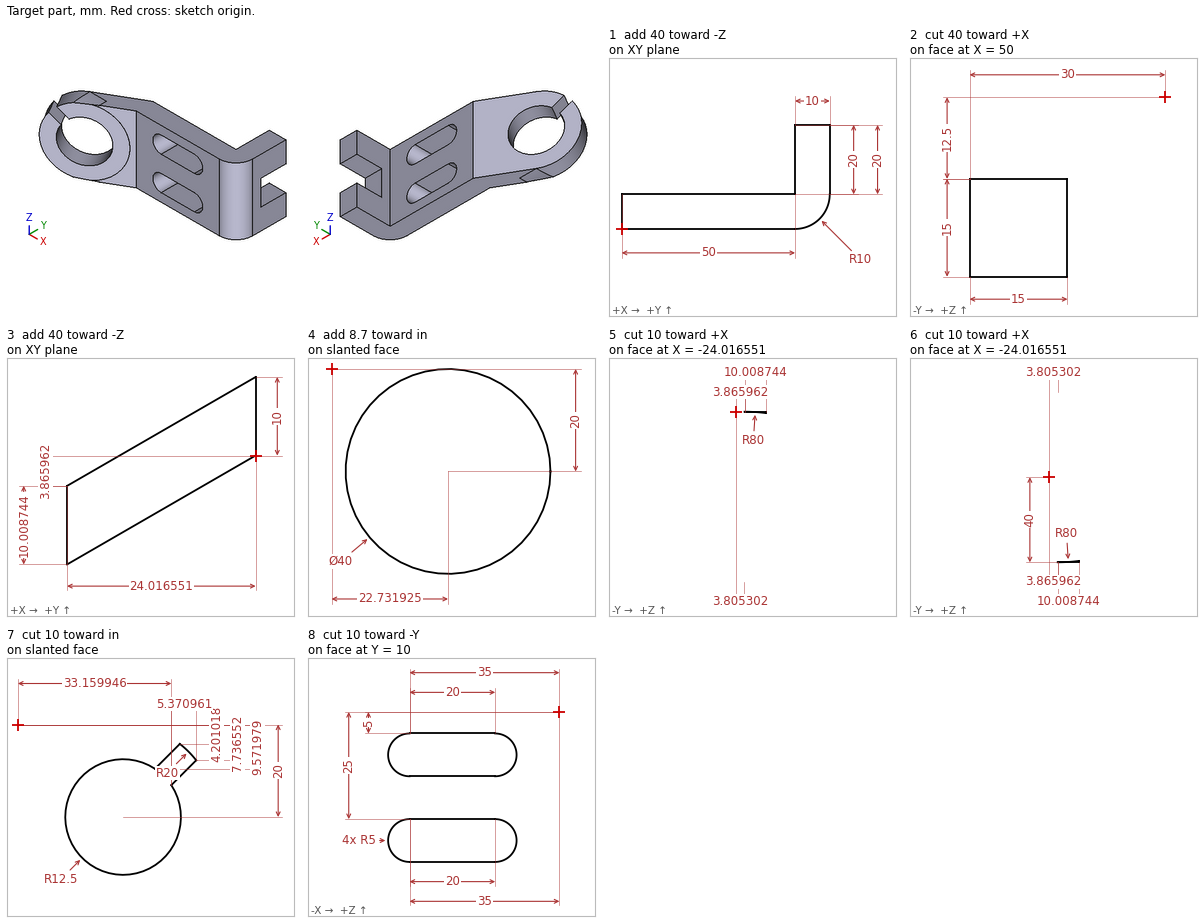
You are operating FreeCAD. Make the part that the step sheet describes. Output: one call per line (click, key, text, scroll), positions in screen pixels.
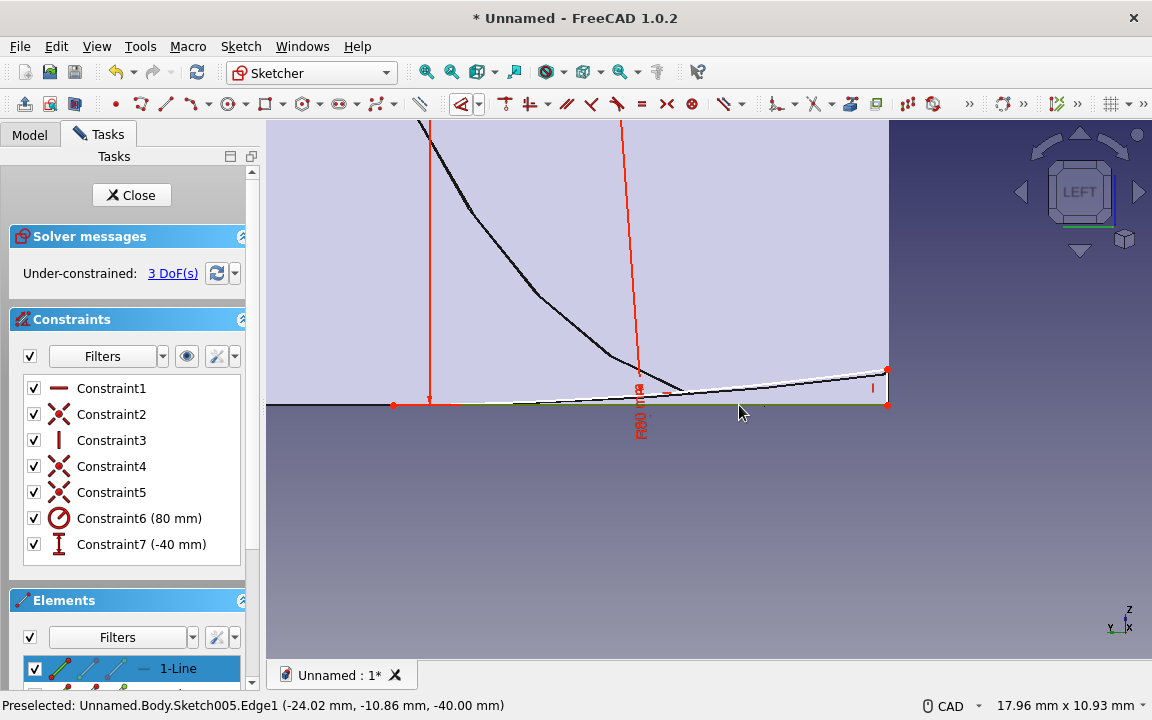
key(l)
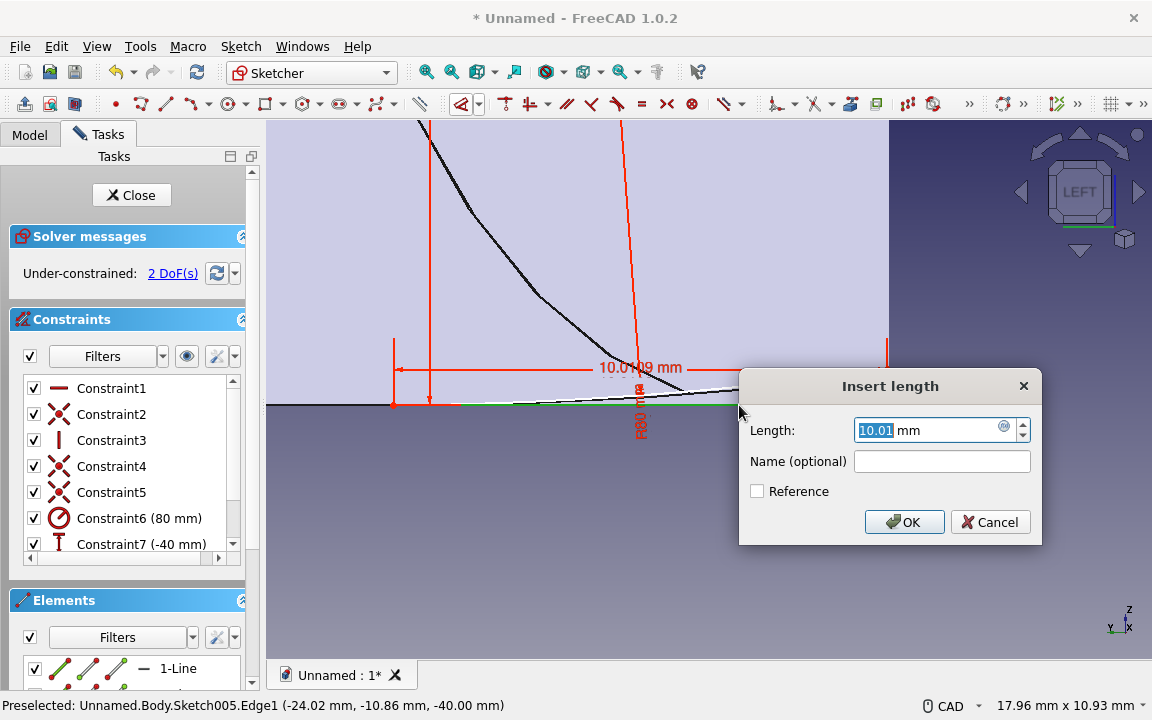
text(10.008744)
key(Return)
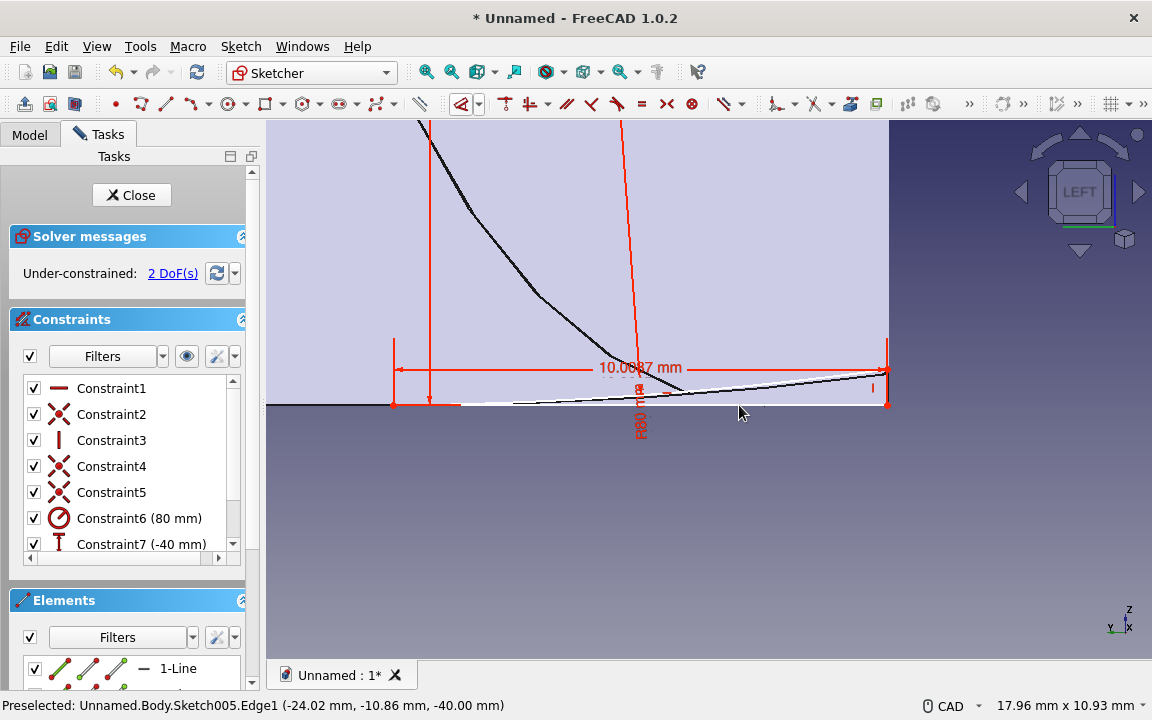
click(394, 405)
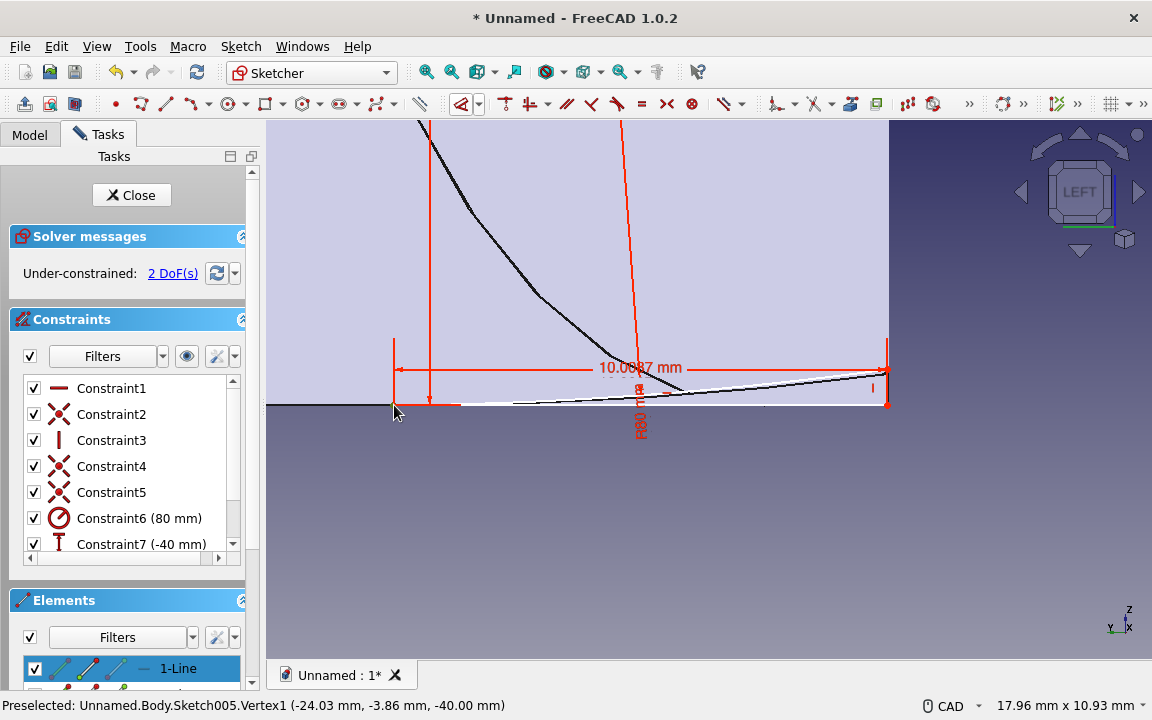
click(478, 104)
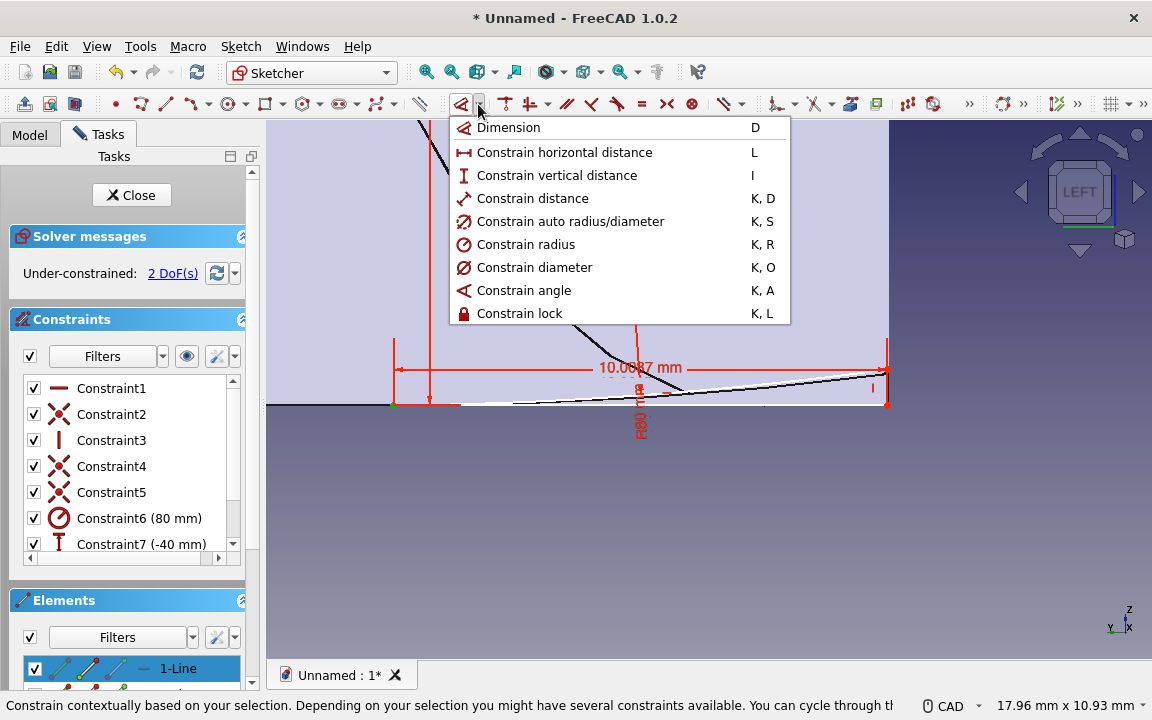
click(620, 152)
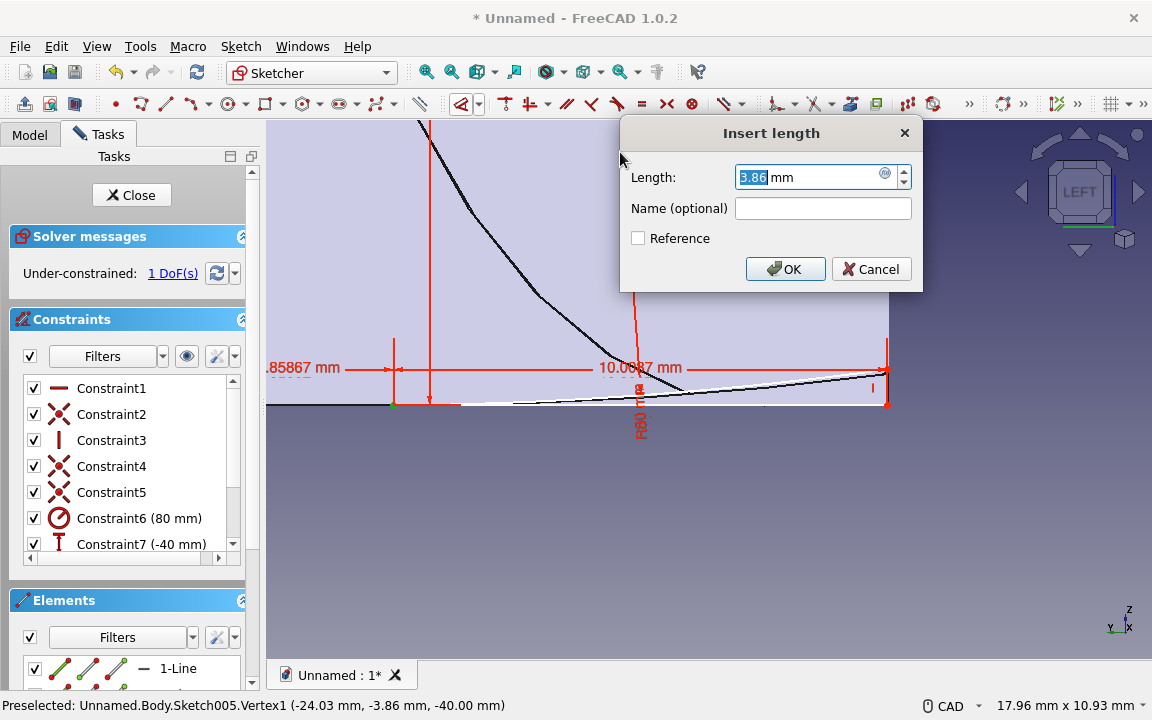
text(3.865962)
key(Return)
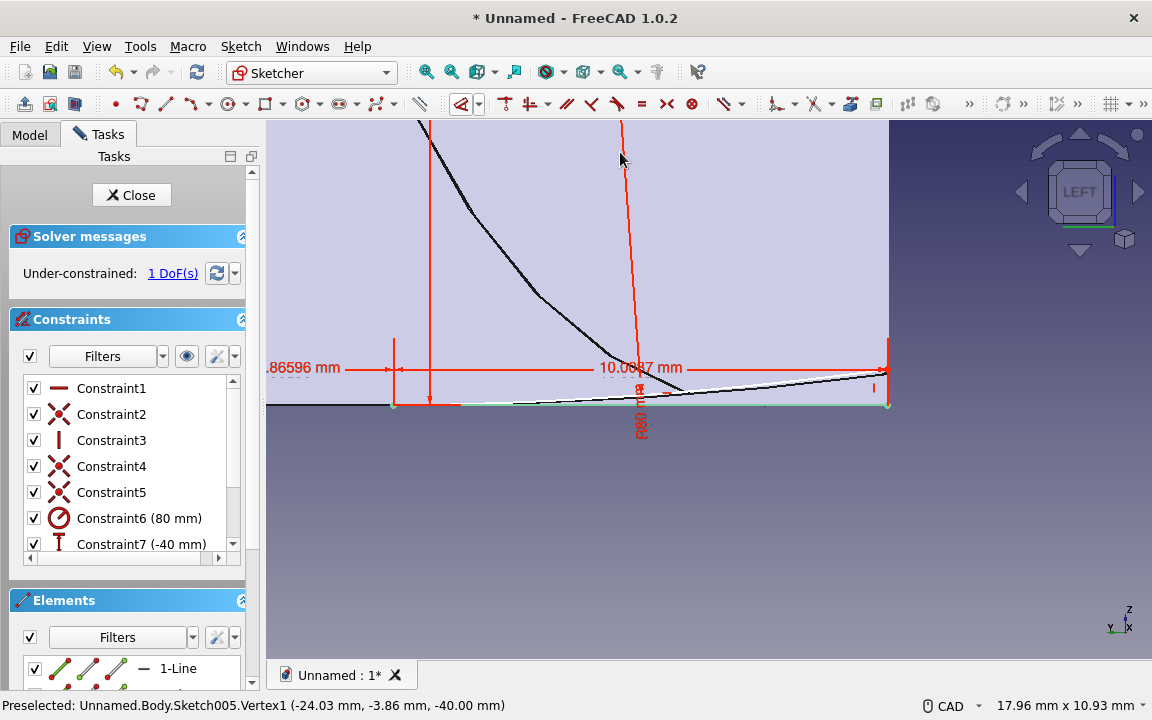
scroll(642, 585, down, 12)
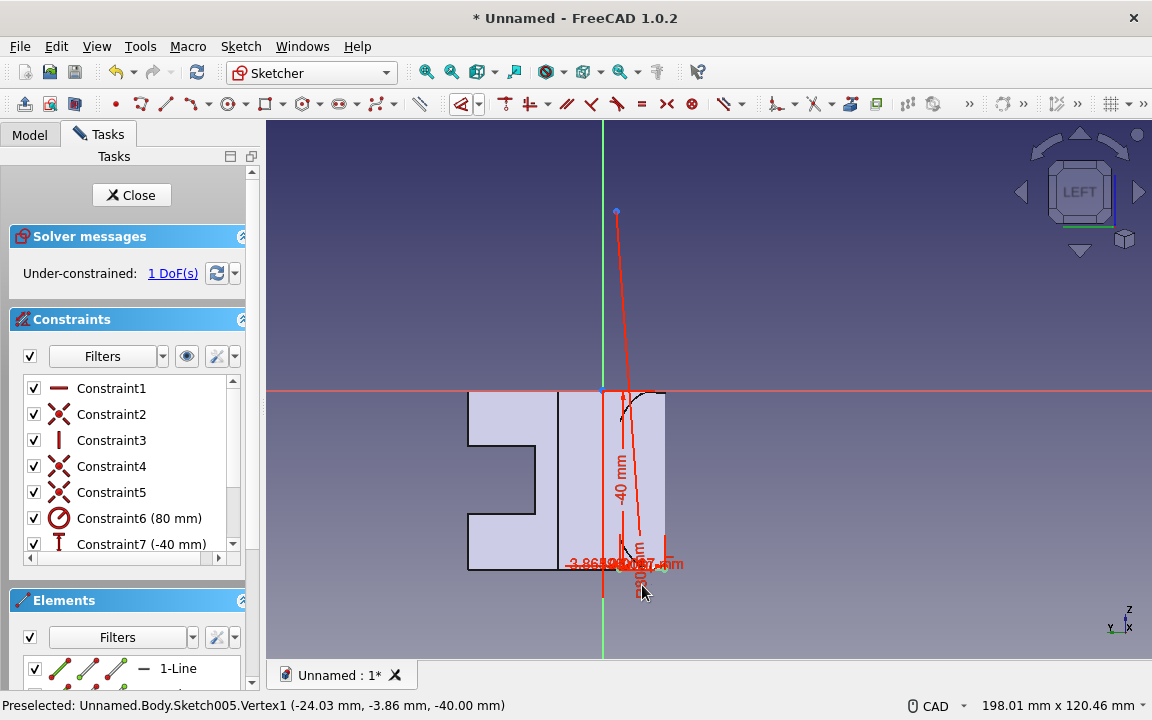
scroll(616, 212, up, 5)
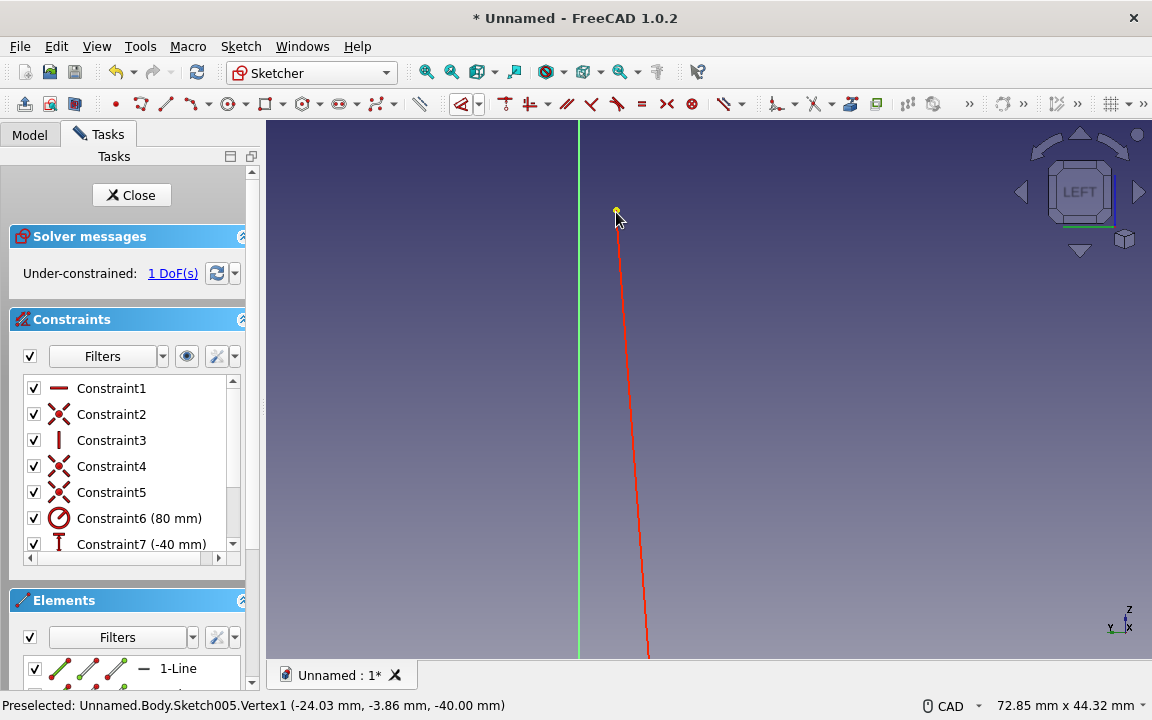
click(616, 211)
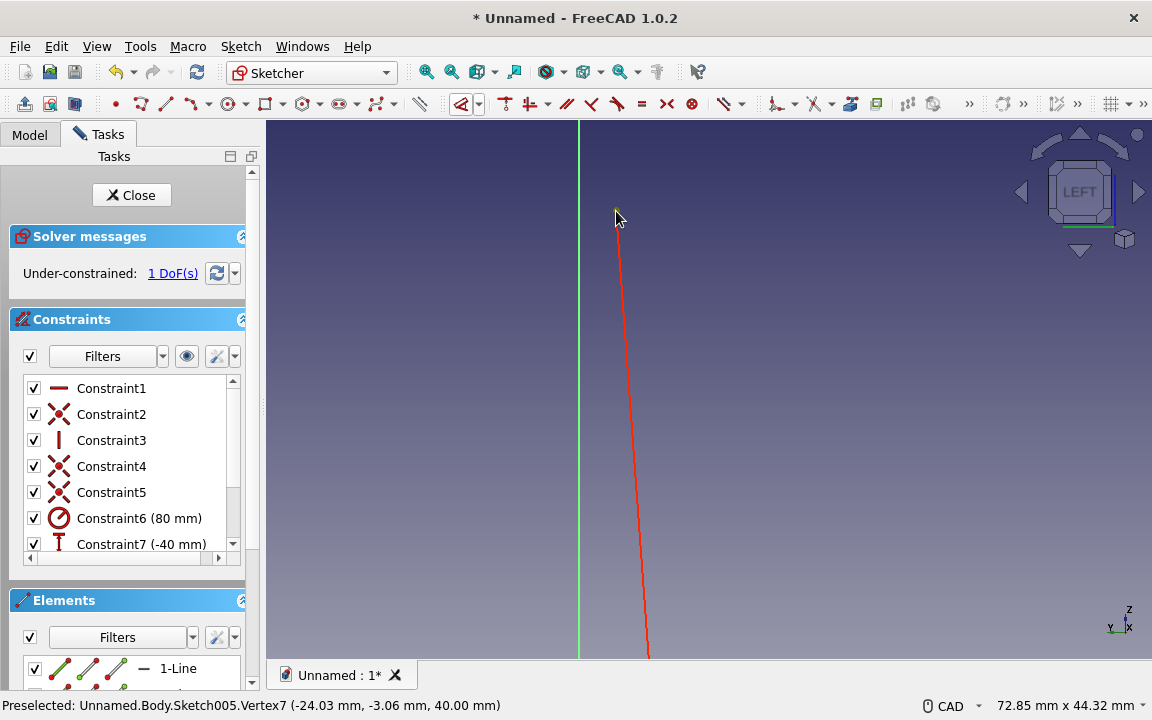
click(478, 104)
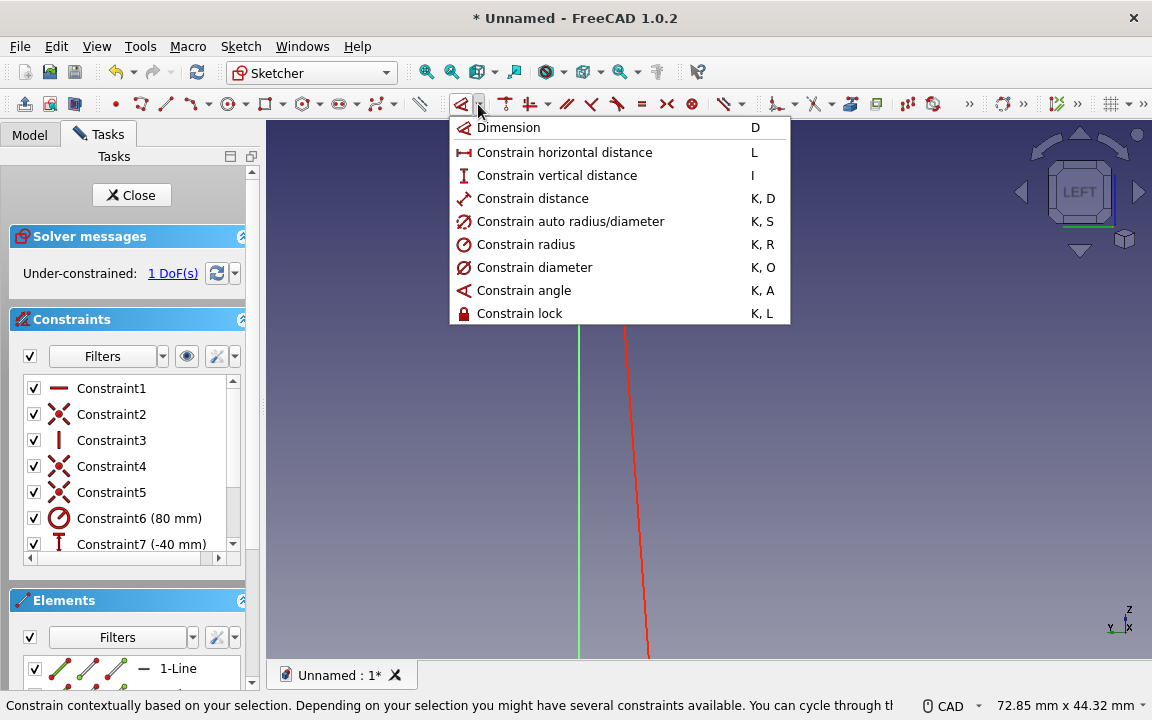
click(620, 152)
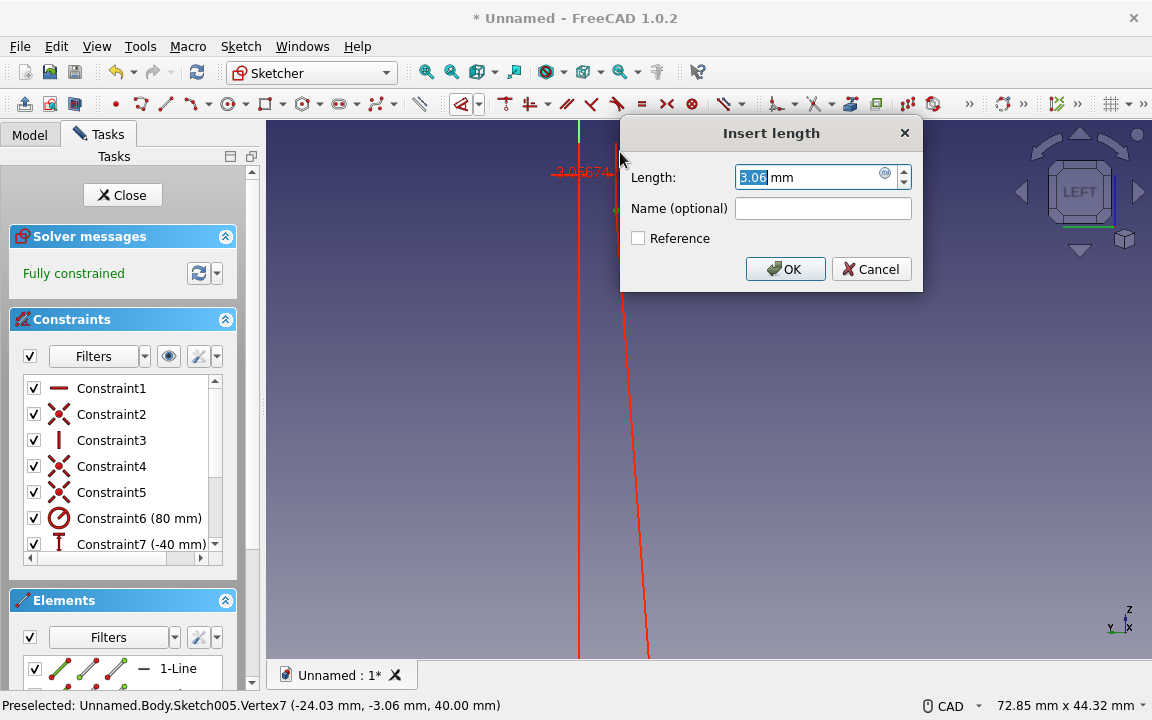
text(3.805302)
key(Return)